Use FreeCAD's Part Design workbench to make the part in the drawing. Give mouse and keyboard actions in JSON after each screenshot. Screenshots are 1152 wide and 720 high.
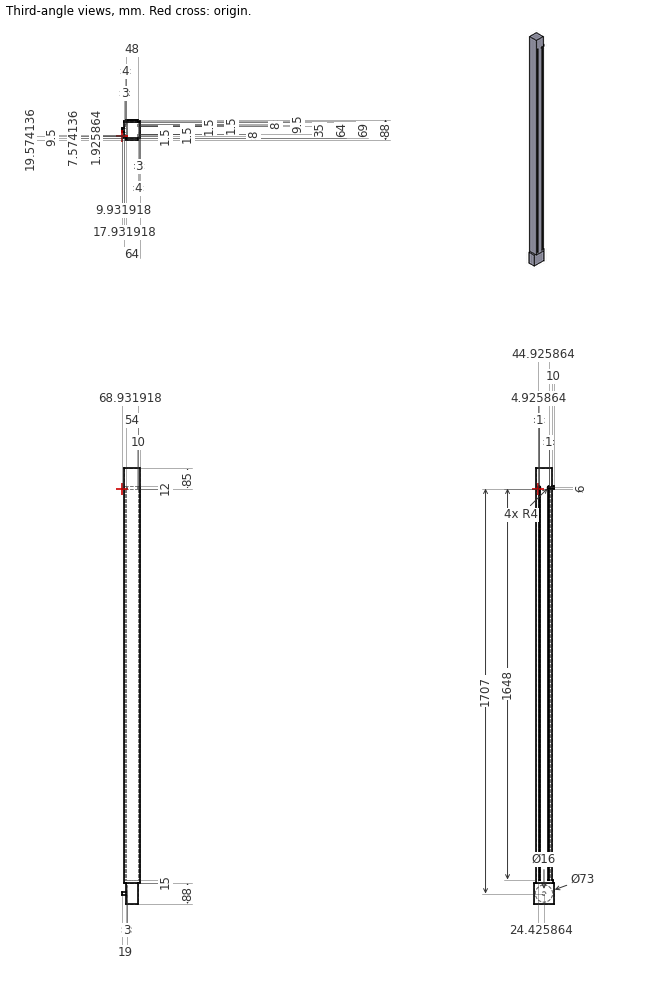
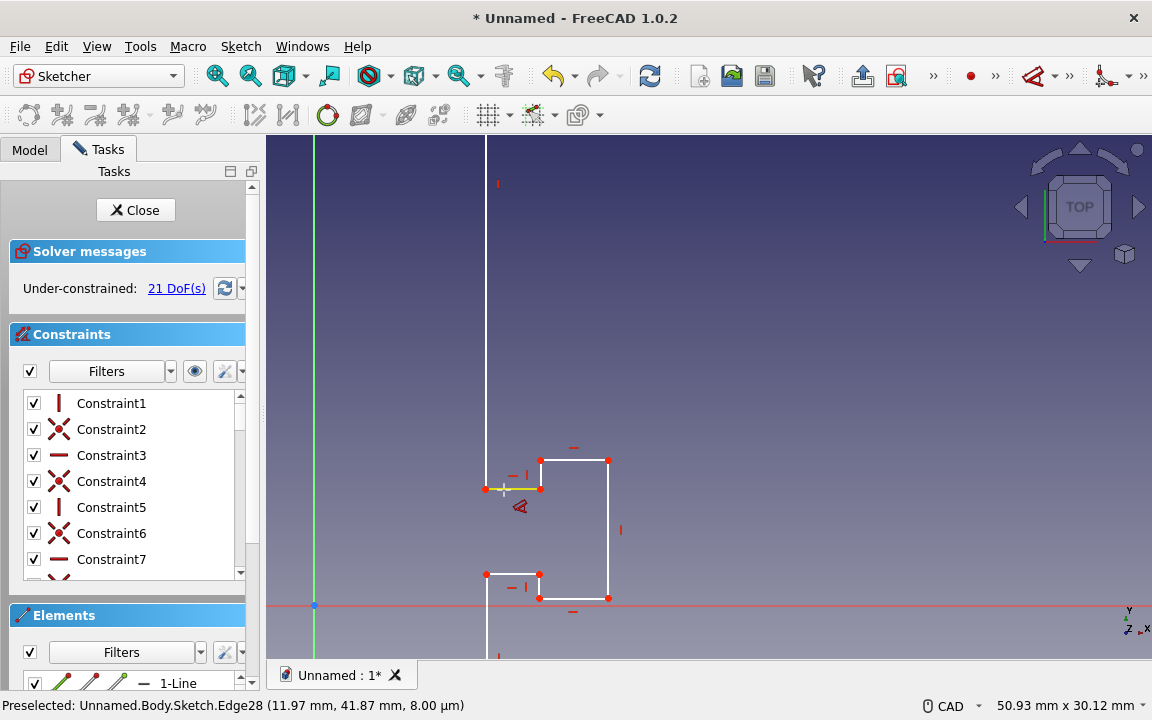
{"action": "left_click", "coordinate": [502, 489]}
{"action": "left_click", "coordinate": [513, 523]}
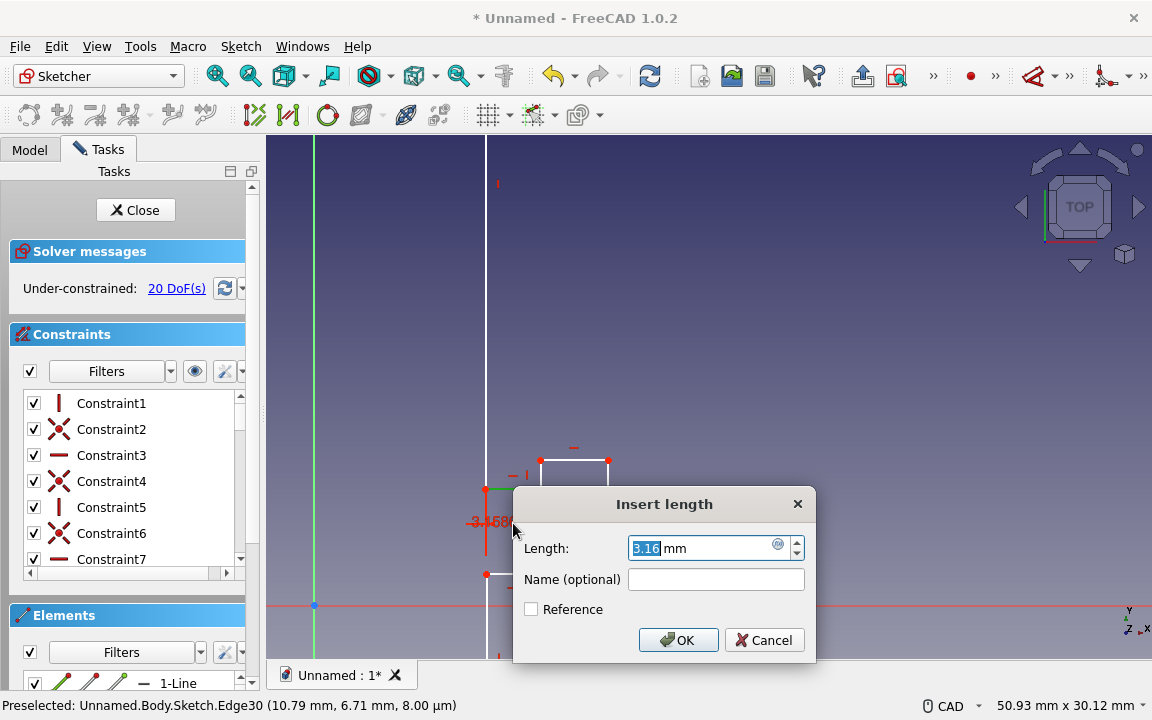
{"action": "type", "text": "3"}
{"action": "key", "text": "Return"}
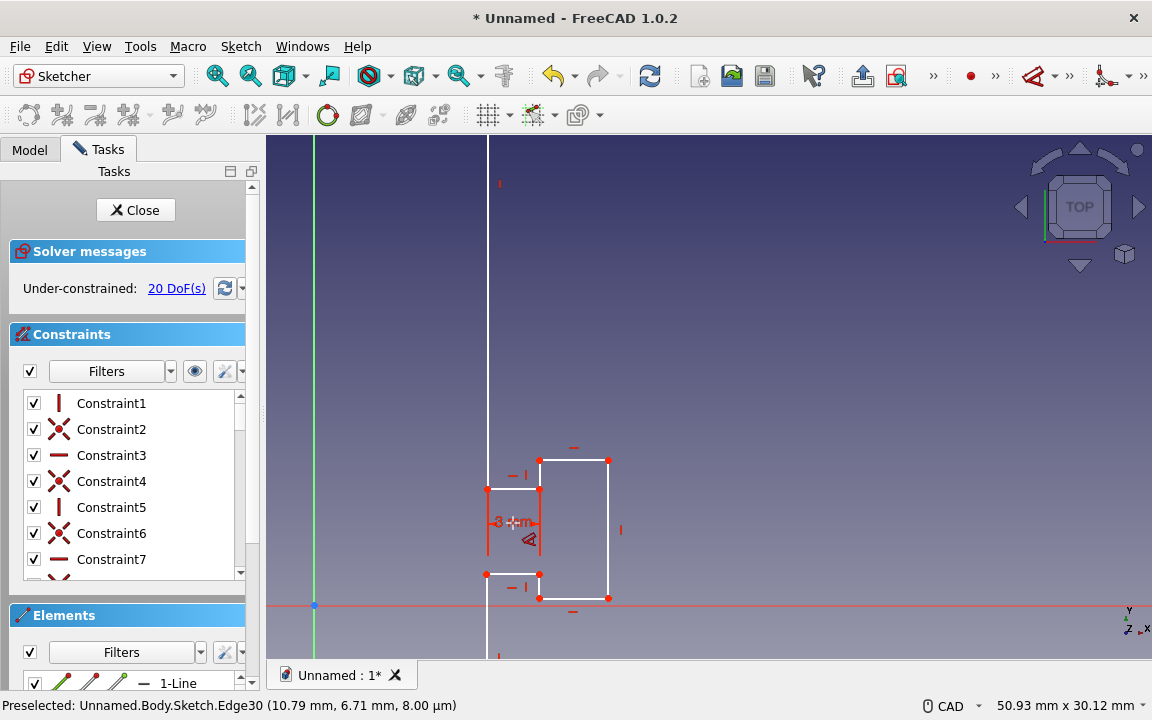
{"action": "left_click", "coordinate": [560, 460]}
{"action": "left_click", "coordinate": [574, 494]}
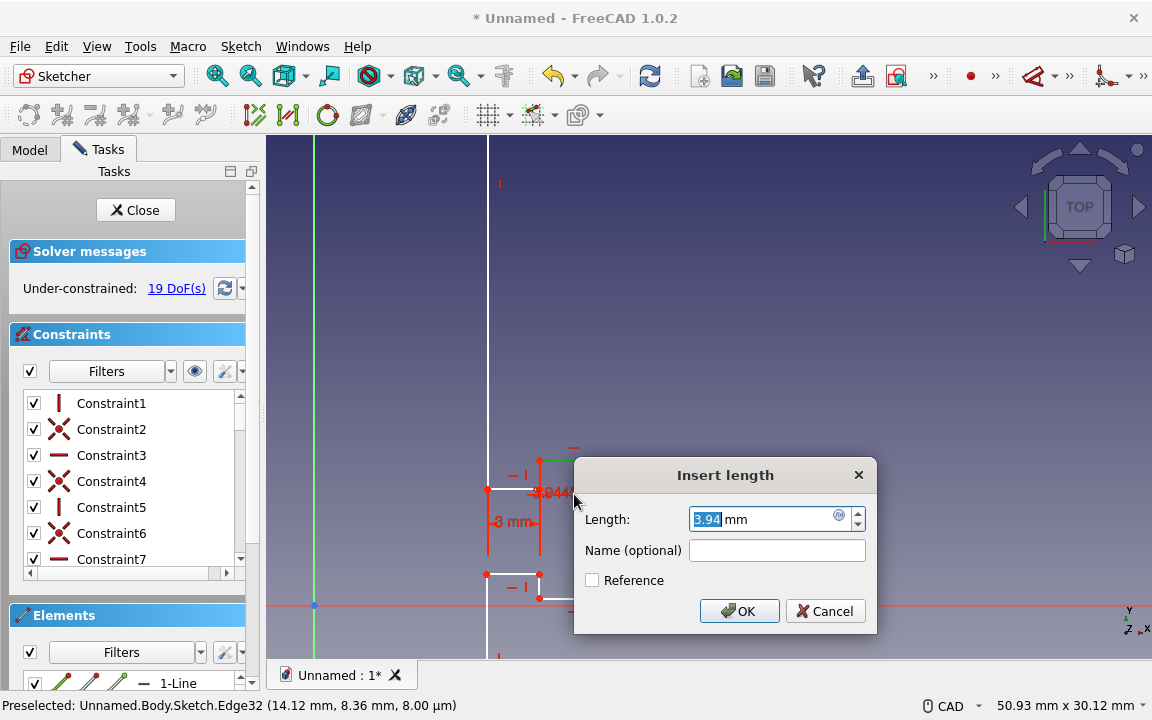
{"action": "type", "text": "4"}
{"action": "key", "text": "Return"}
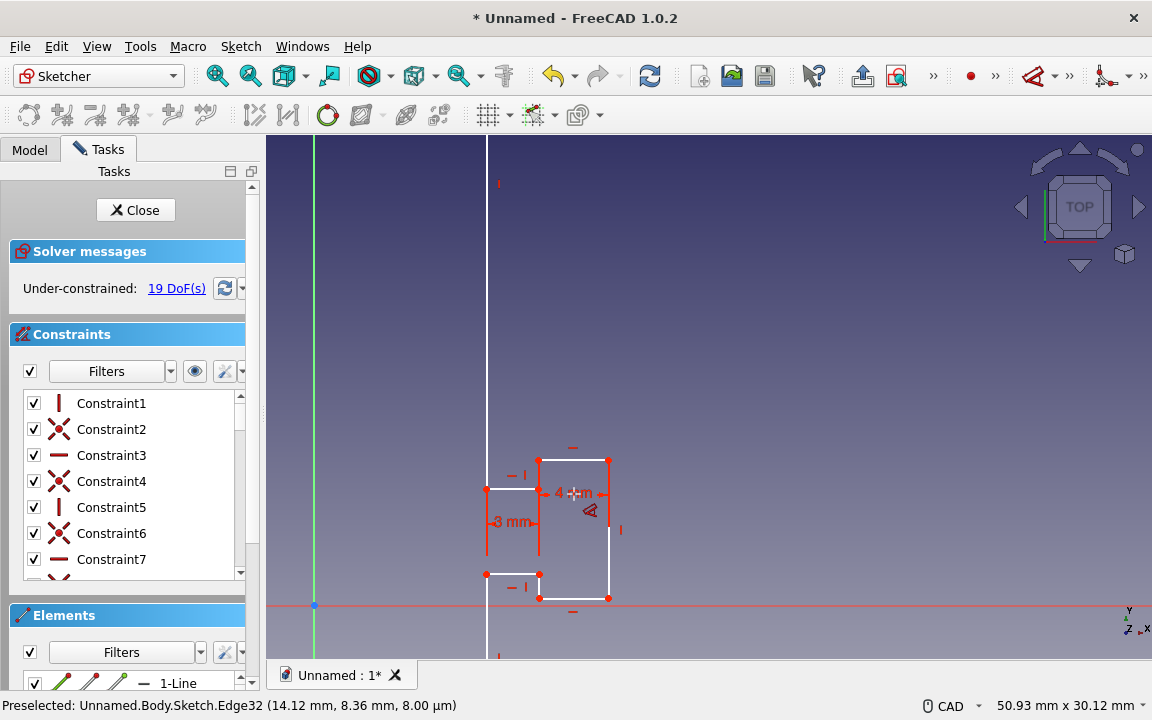
{"action": "scroll", "coordinate": [504, 490], "scroll_direction": "down", "scroll_amount": 6}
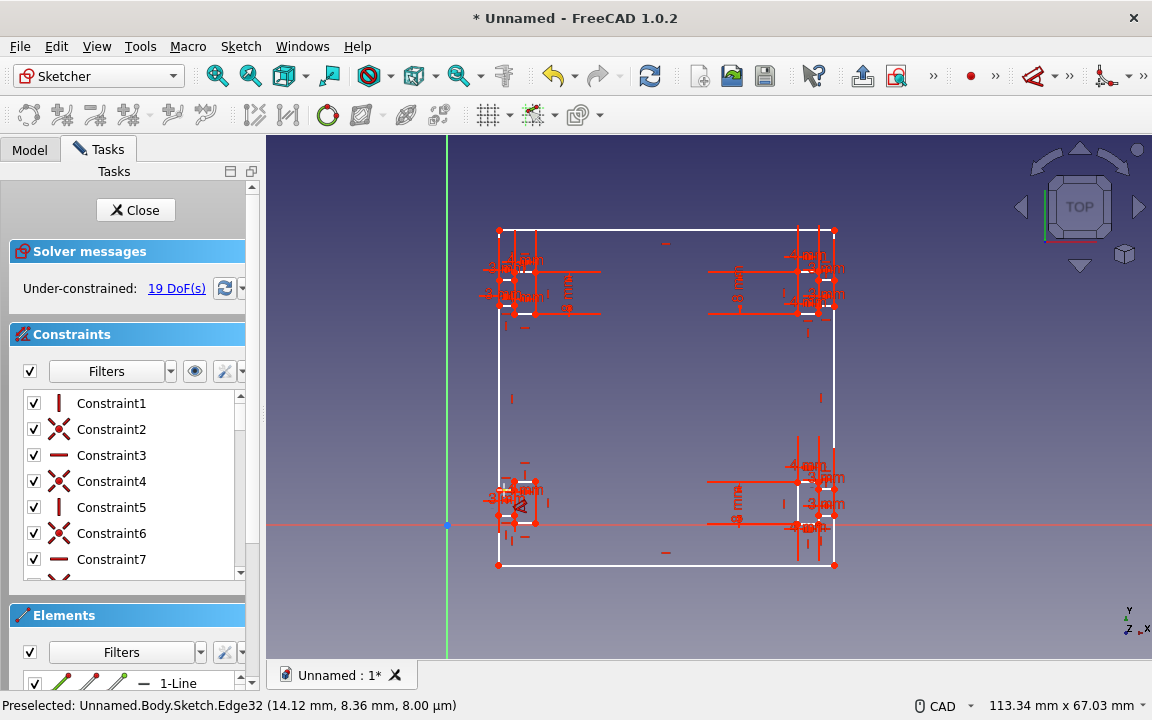
{"action": "left_click", "coordinate": [536, 494]}
{"action": "left_click", "coordinate": [594, 512]}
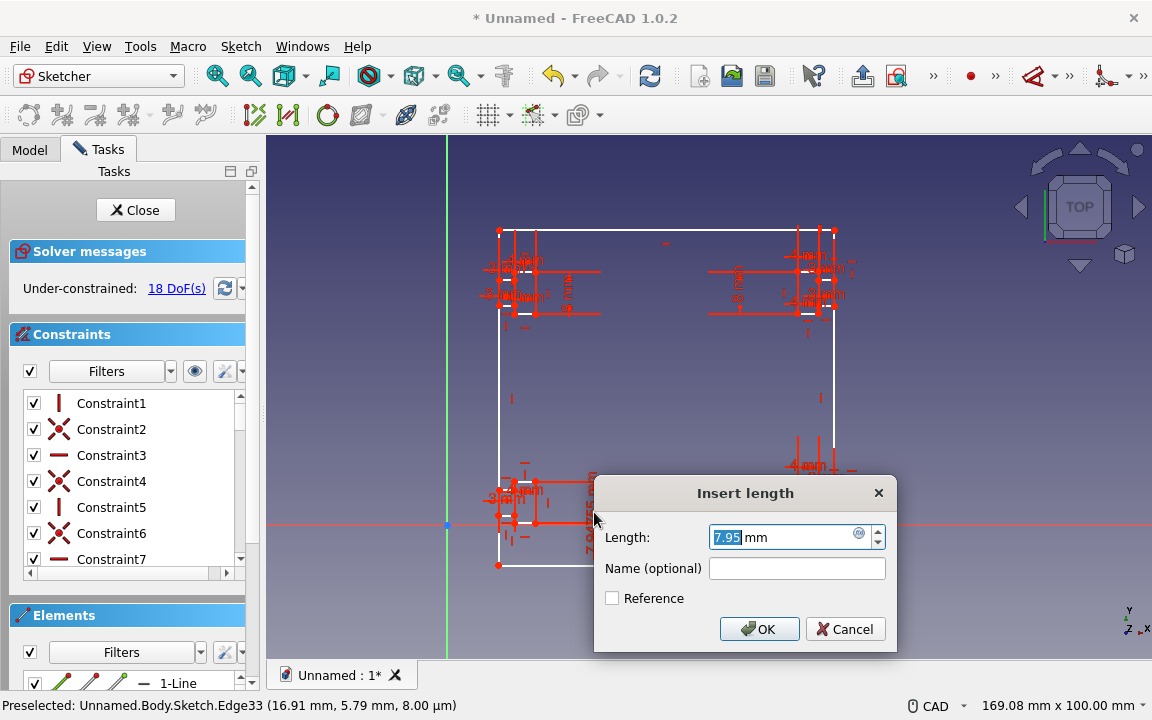
{"action": "type", "text": "8"}
{"action": "key", "text": "Return"}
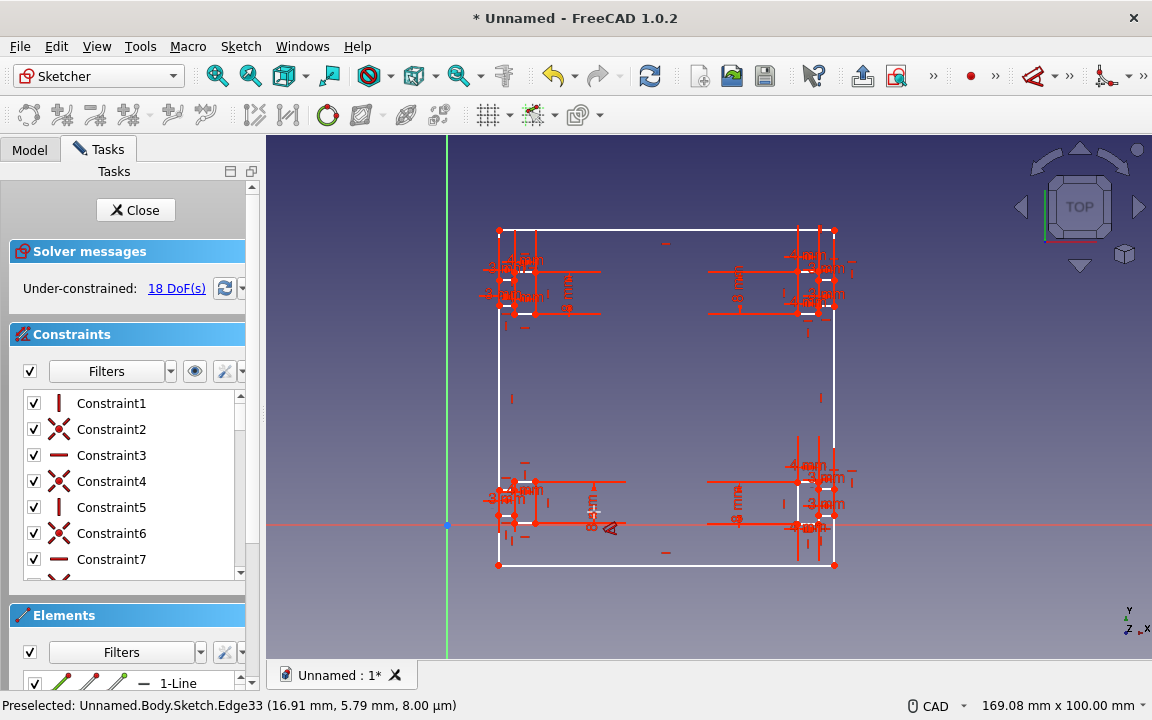
{"action": "scroll", "coordinate": [525, 523], "scroll_direction": "up", "scroll_amount": 4}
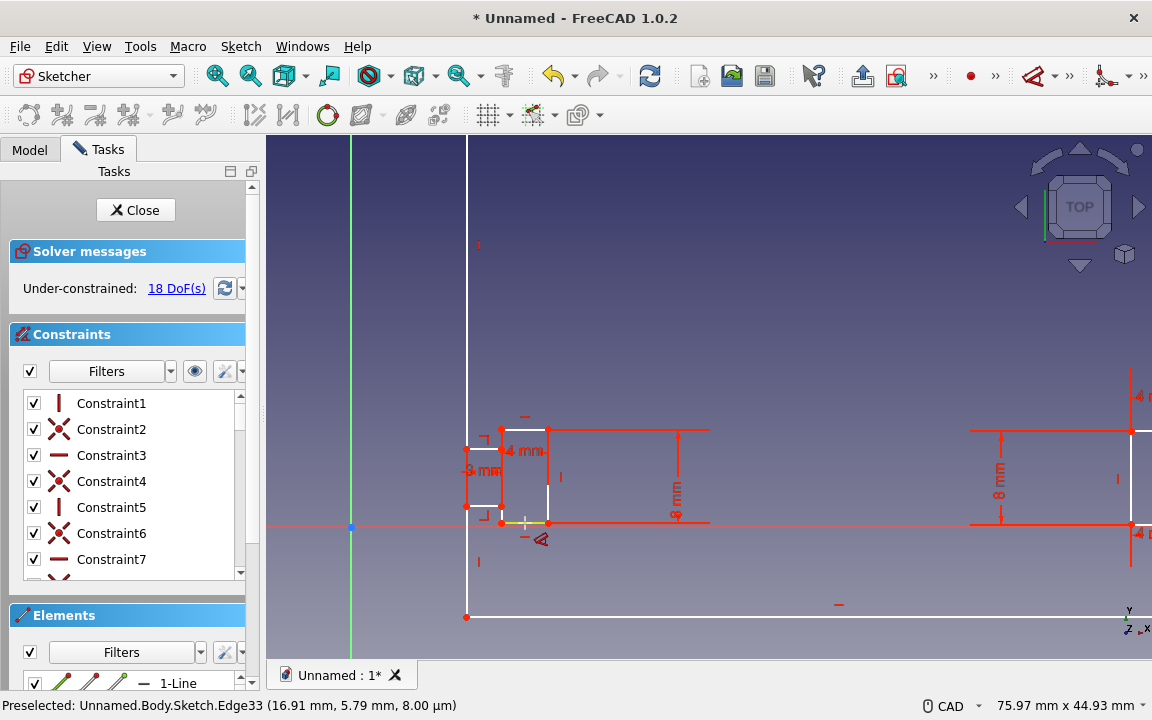
{"action": "left_click", "coordinate": [525, 523]}
{"action": "left_click", "coordinate": [525, 557]}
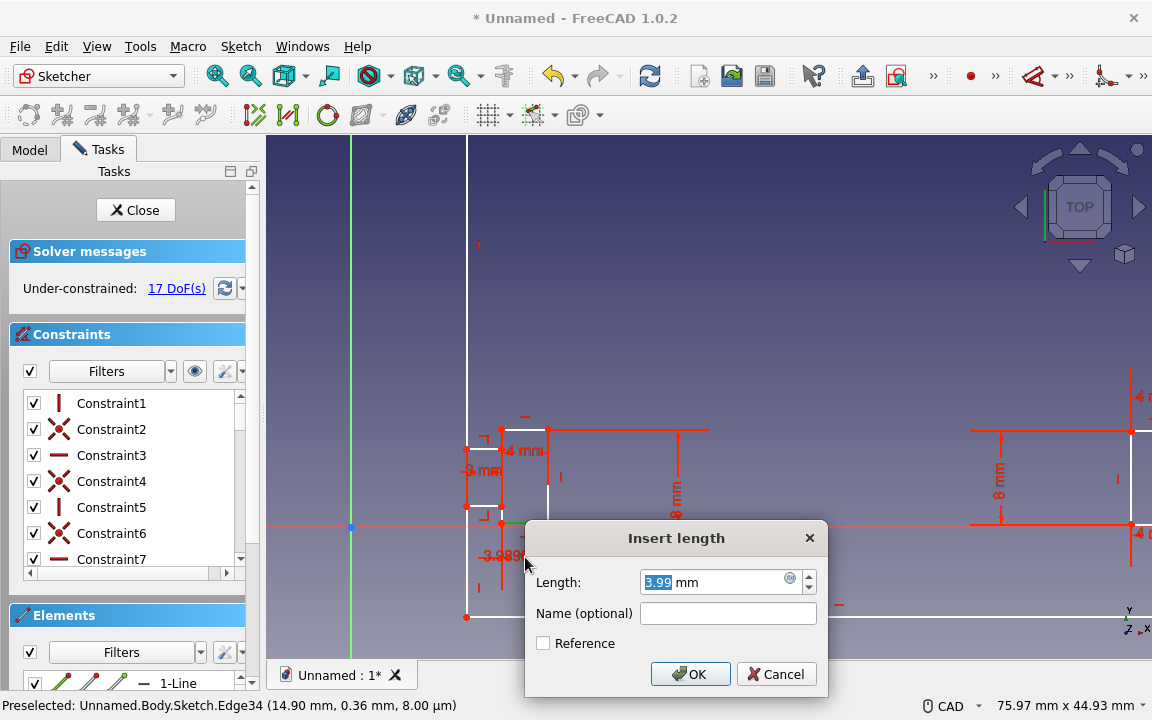
{"action": "type", "text": "4"}
{"action": "key", "text": "Return"}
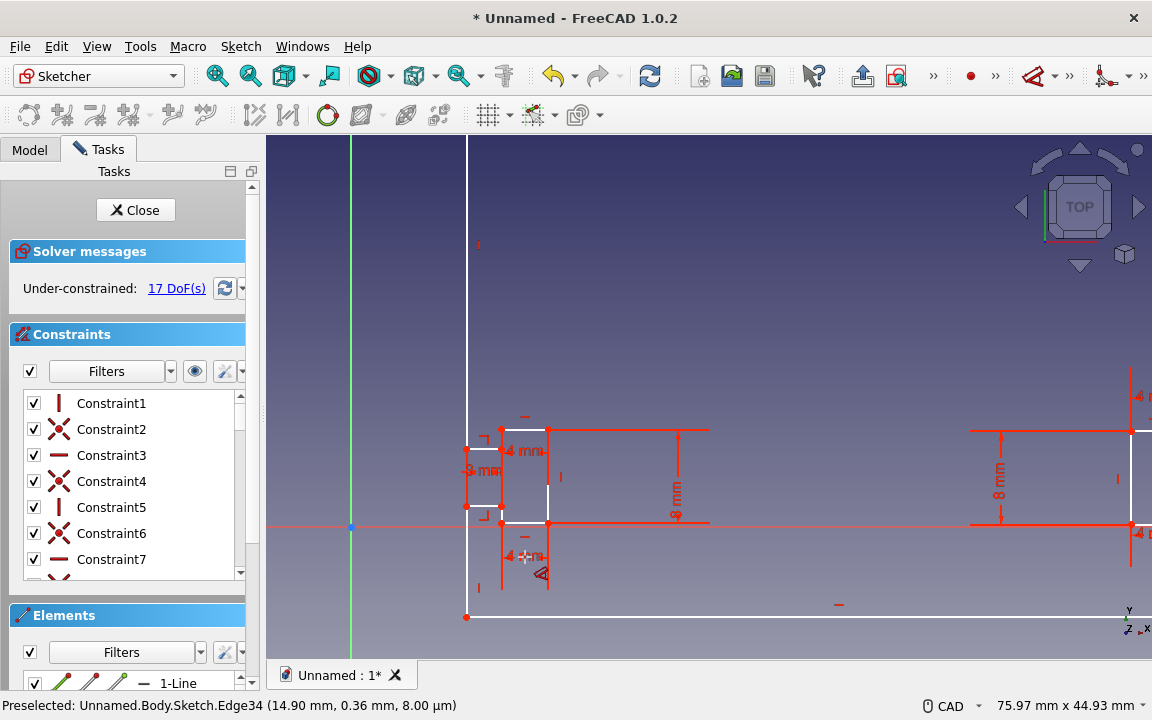
{"action": "scroll", "coordinate": [491, 506], "scroll_direction": "up", "scroll_amount": 2}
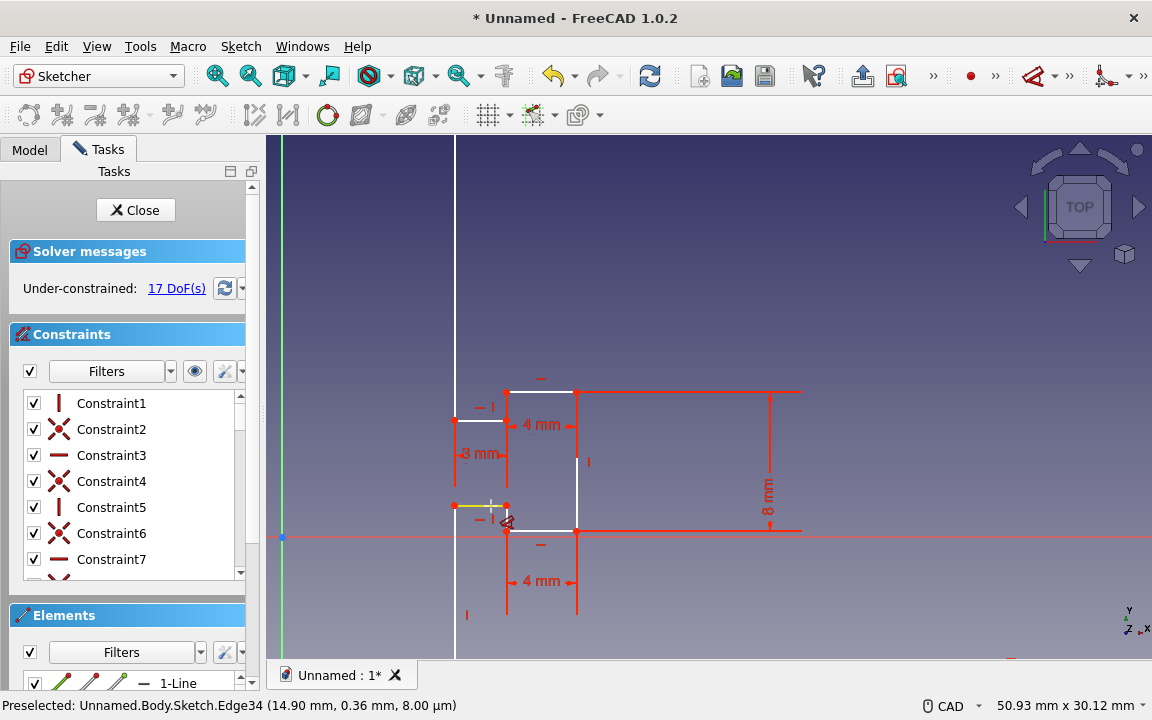
{"action": "left_click", "coordinate": [491, 506]}
{"action": "left_click", "coordinate": [469, 564]}